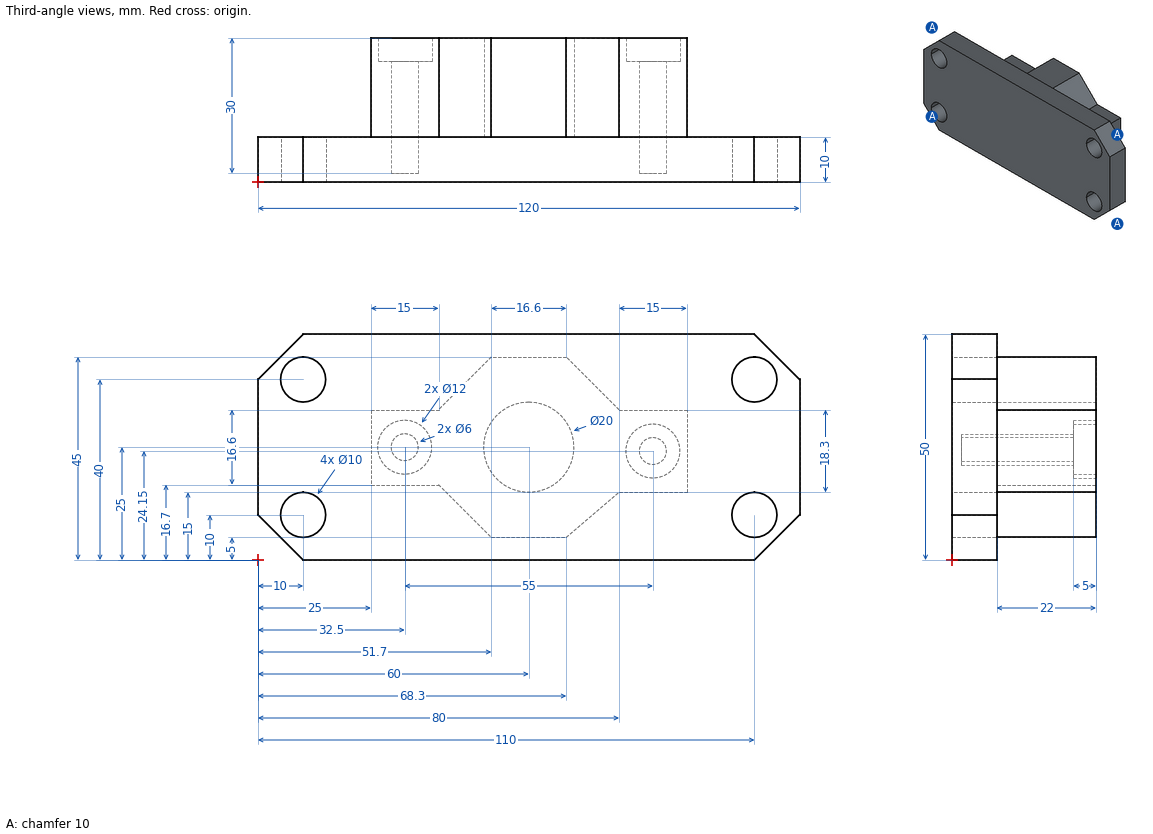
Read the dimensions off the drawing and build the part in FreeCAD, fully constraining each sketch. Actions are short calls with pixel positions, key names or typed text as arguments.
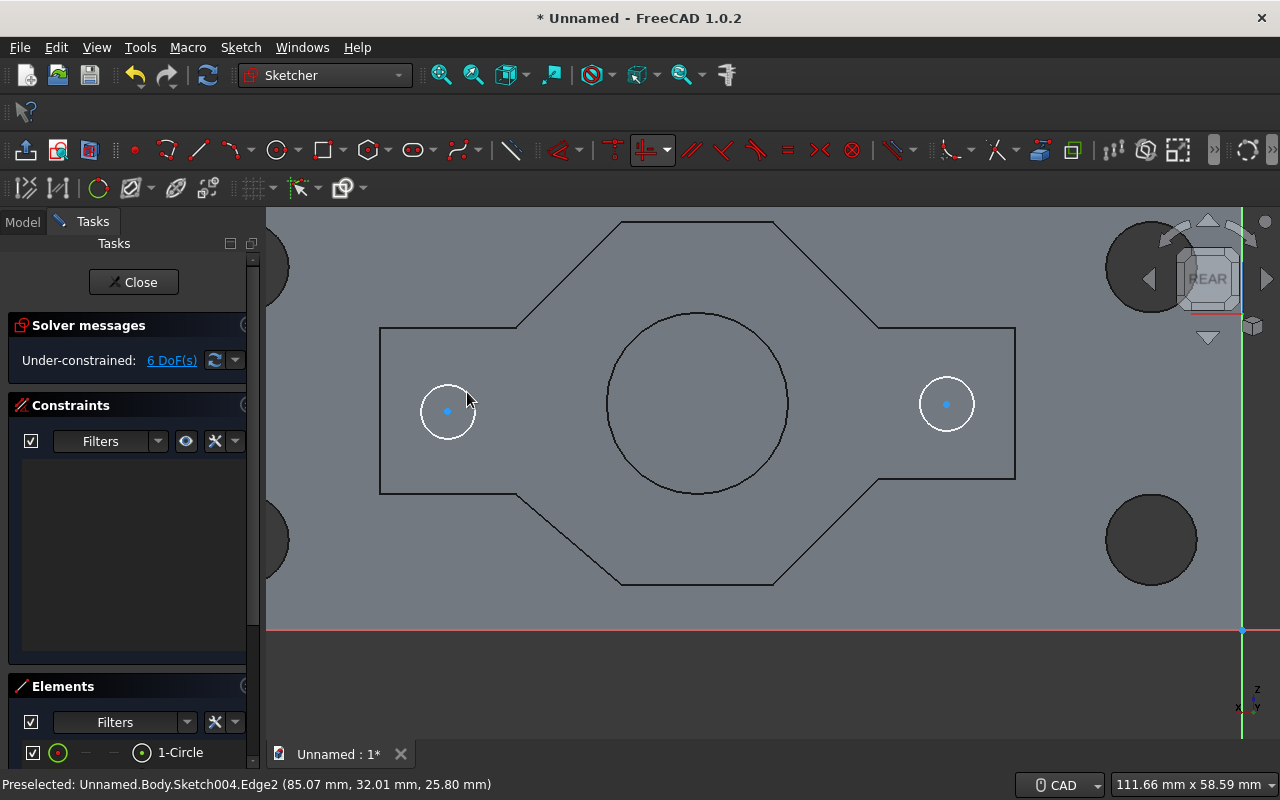
click(966, 385)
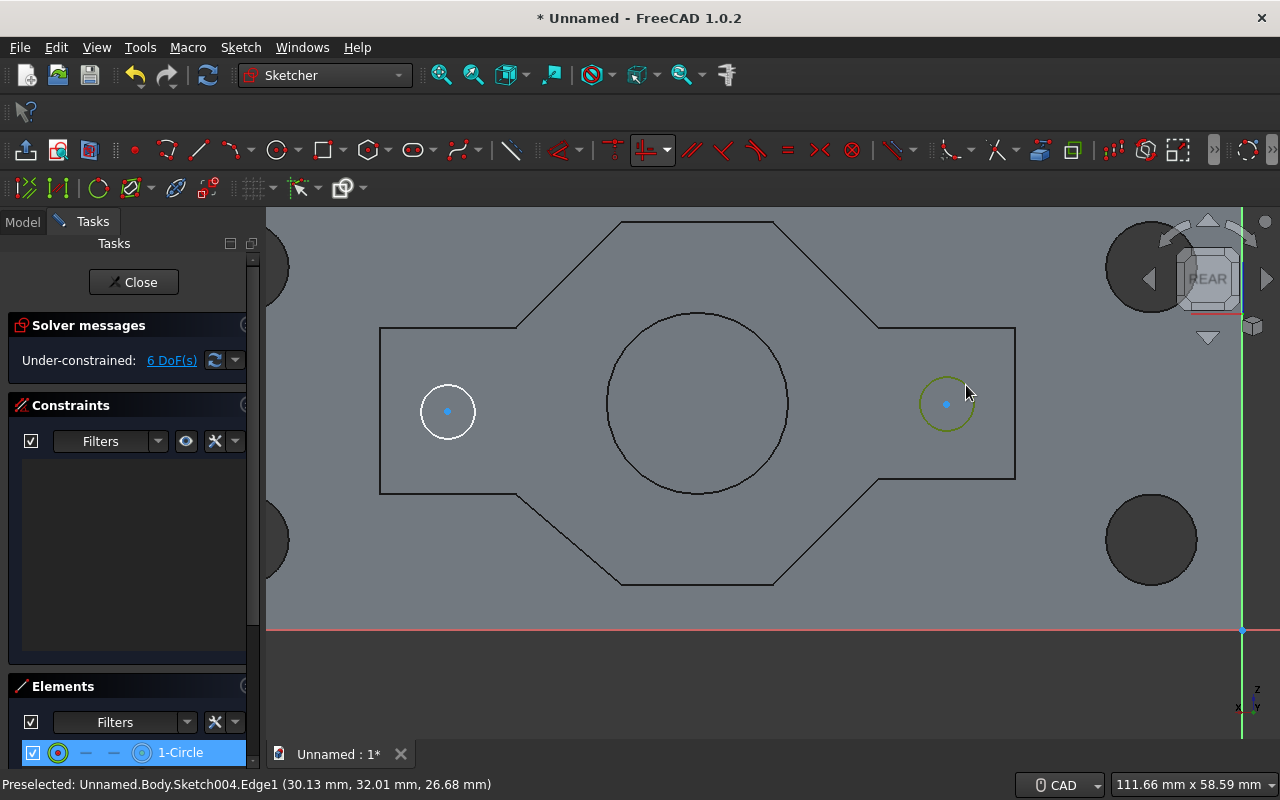
click(467, 393)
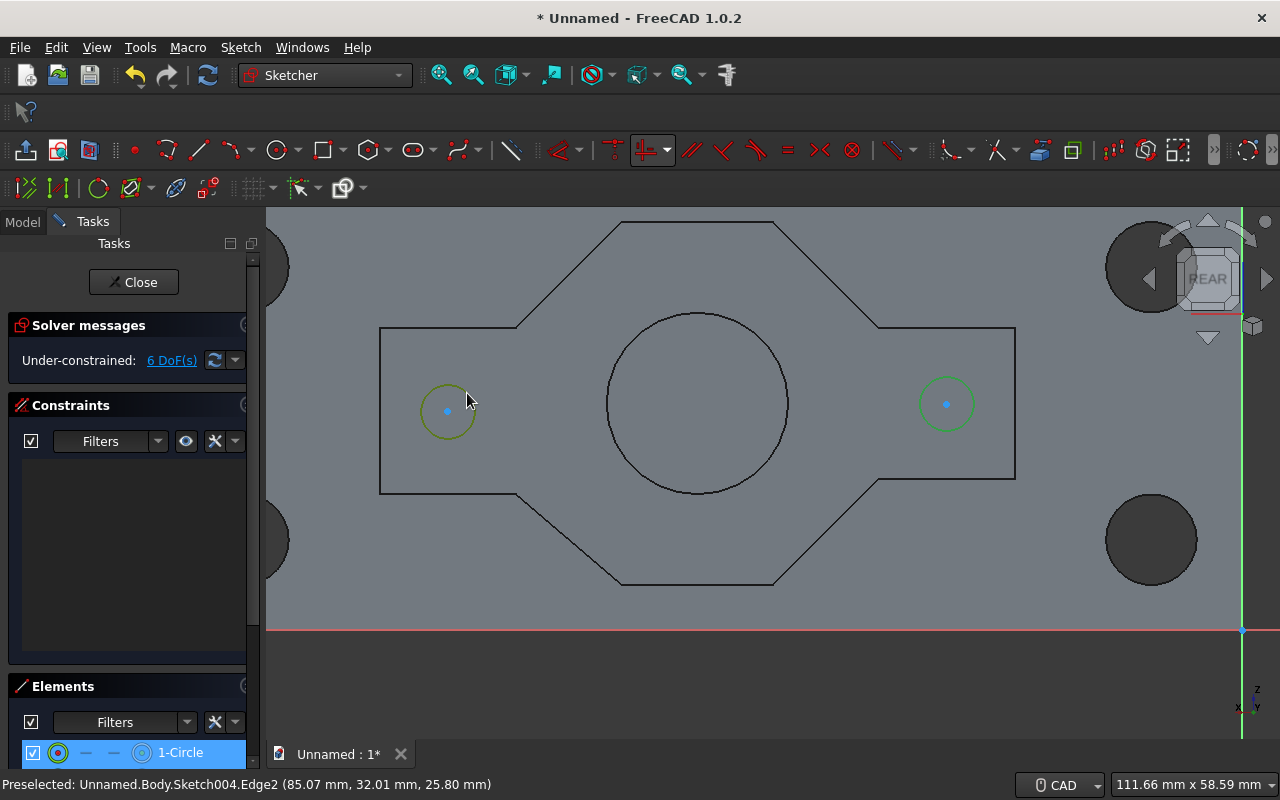
click(788, 150)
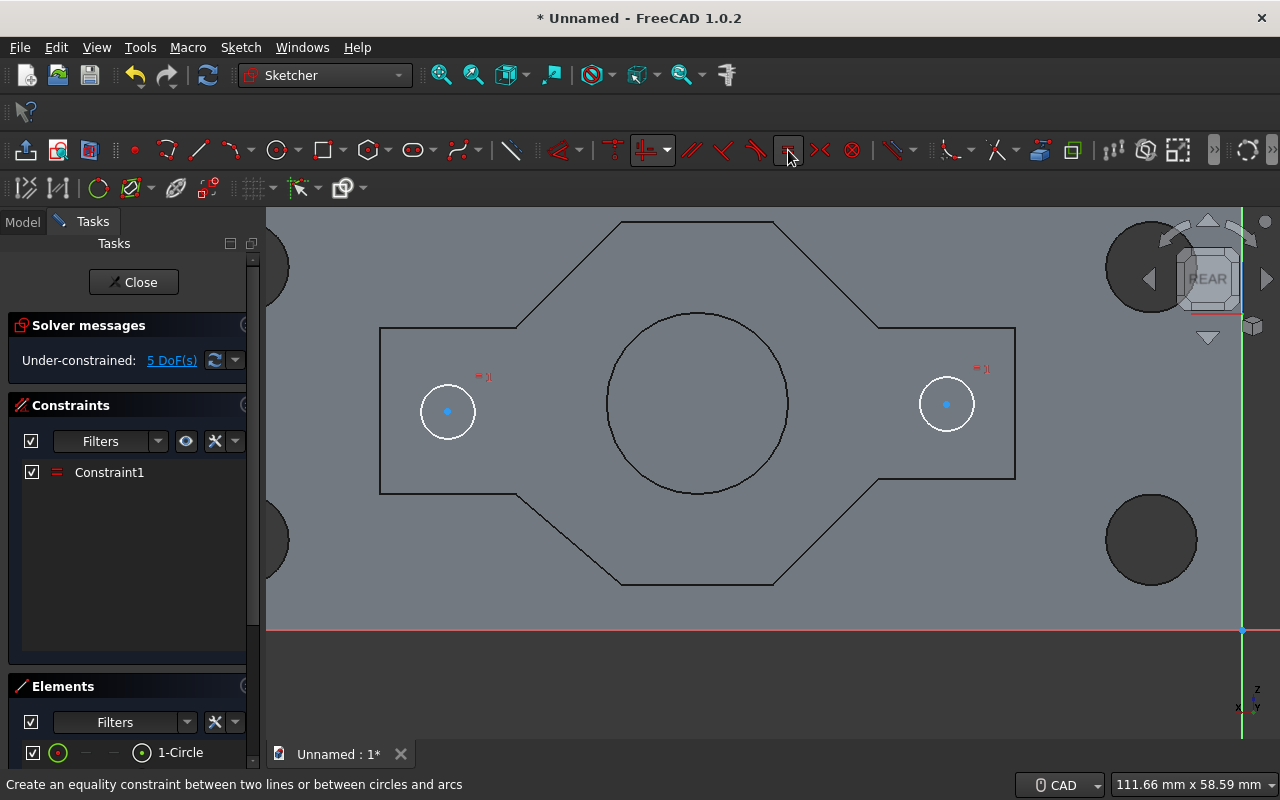
click(558, 150)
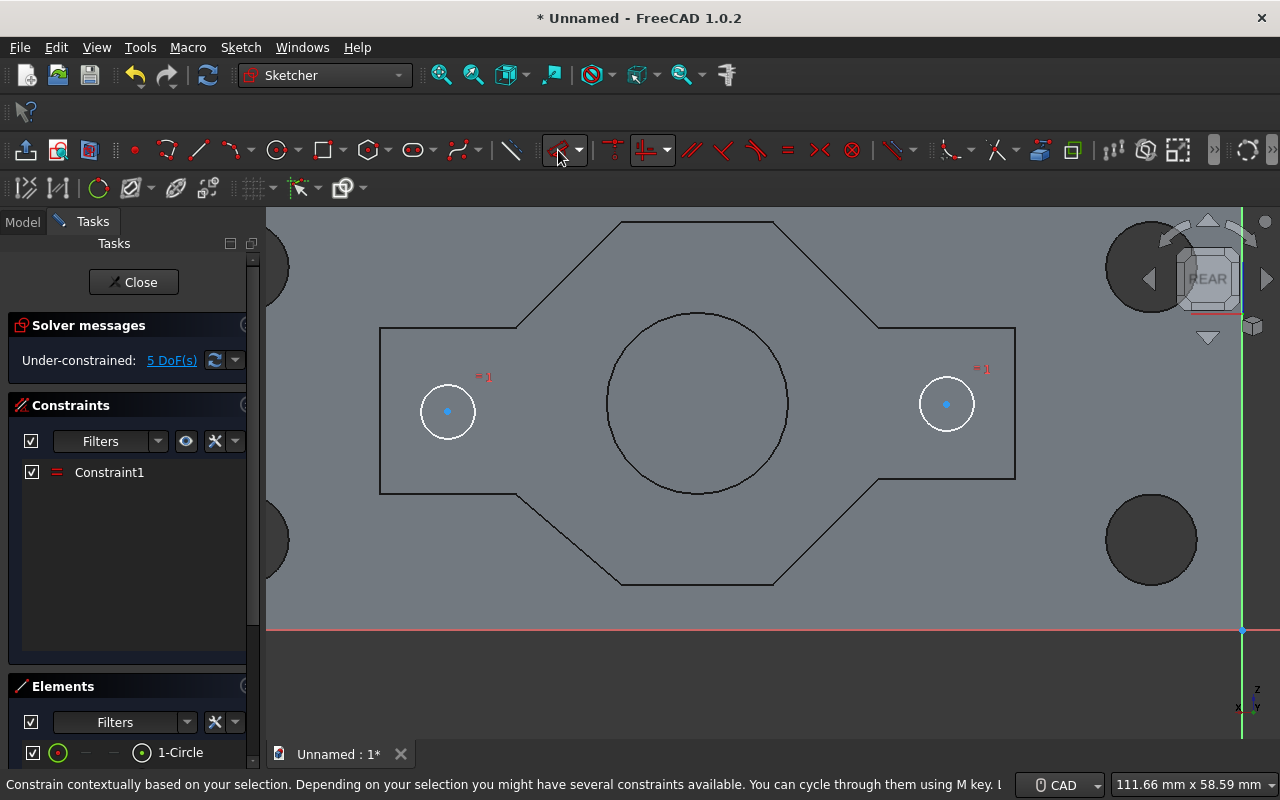
click(966, 385)
click(989, 362)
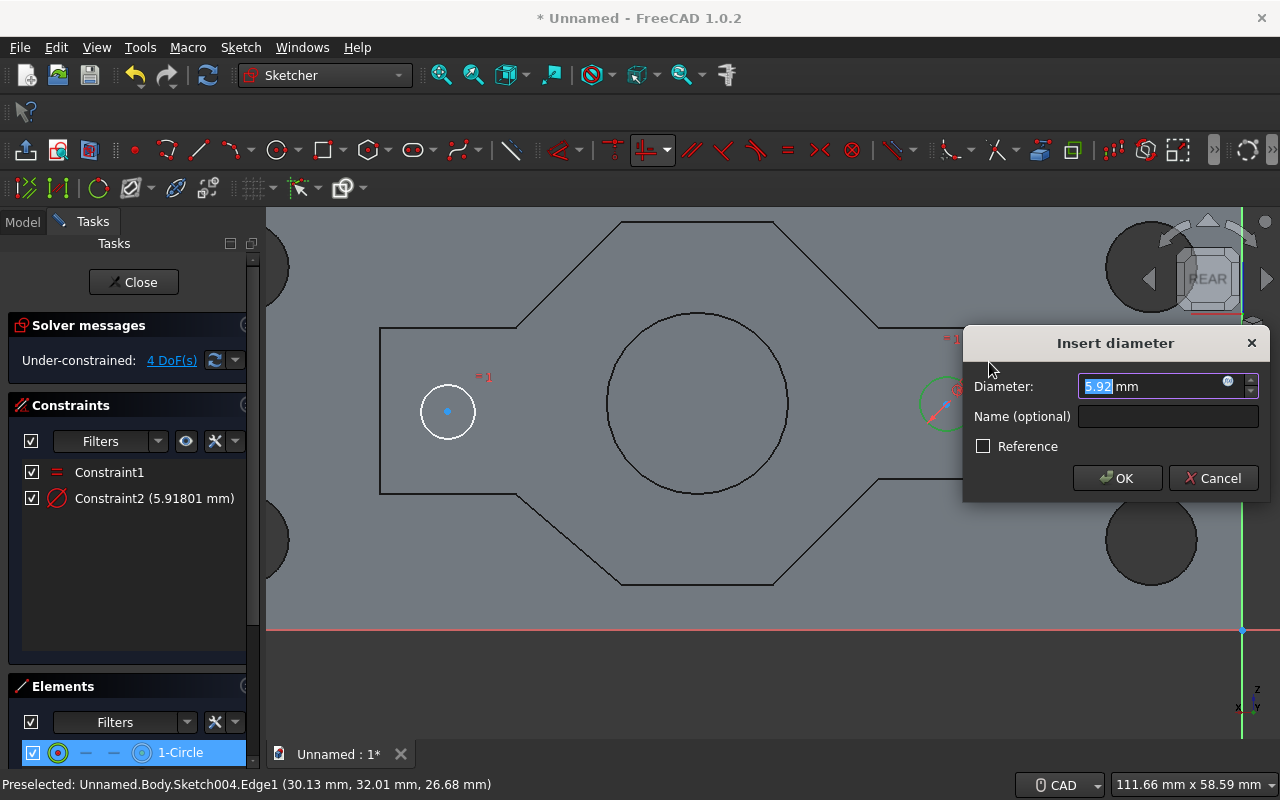
text(6)
key(Return)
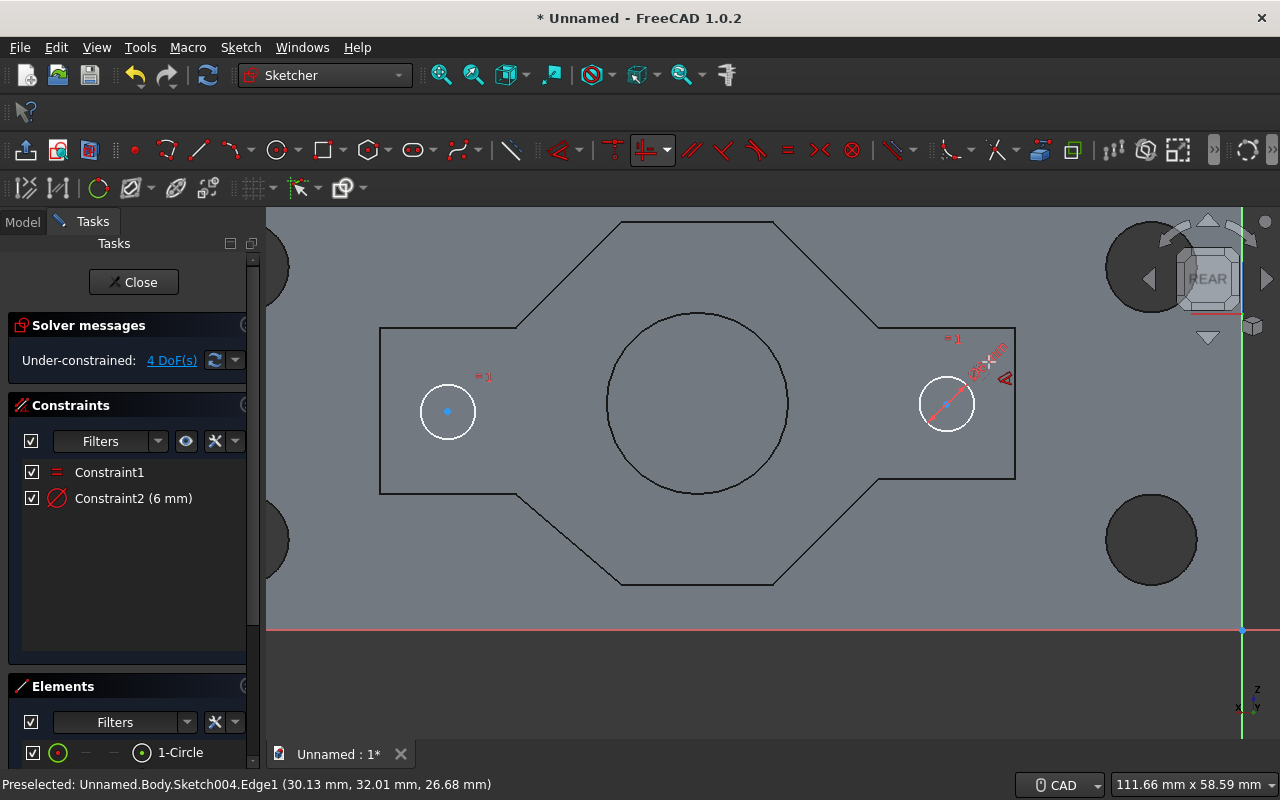
click(947, 404)
click(913, 517)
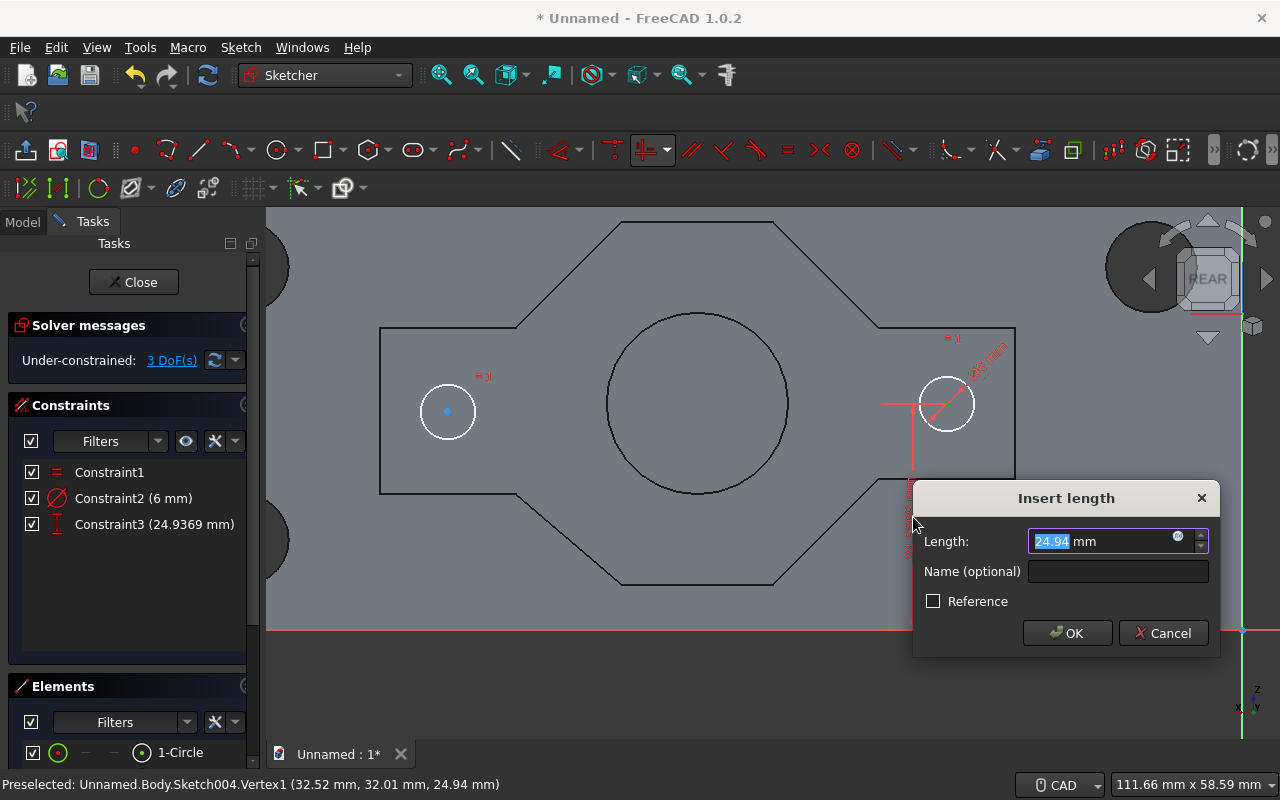
text(25)
key(Return)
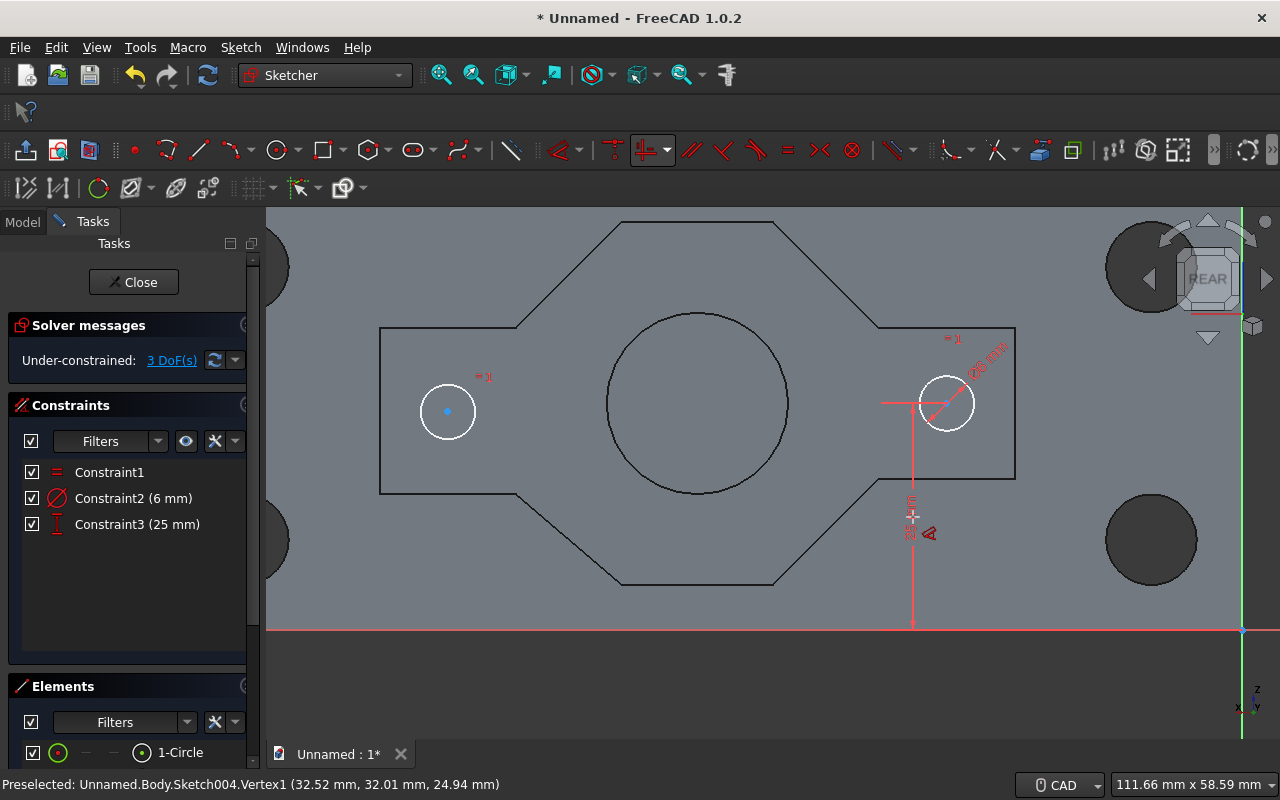
click(947, 403)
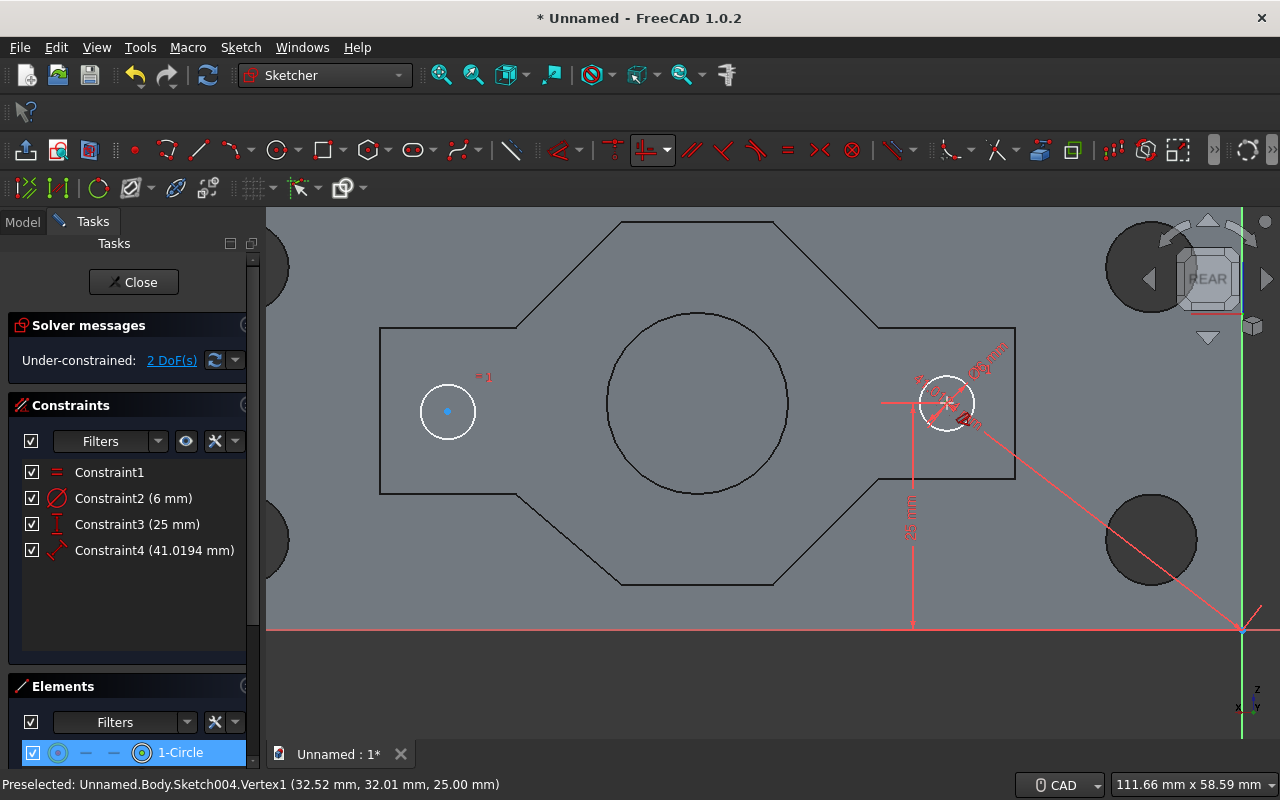
click(448, 412)
click(697, 369)